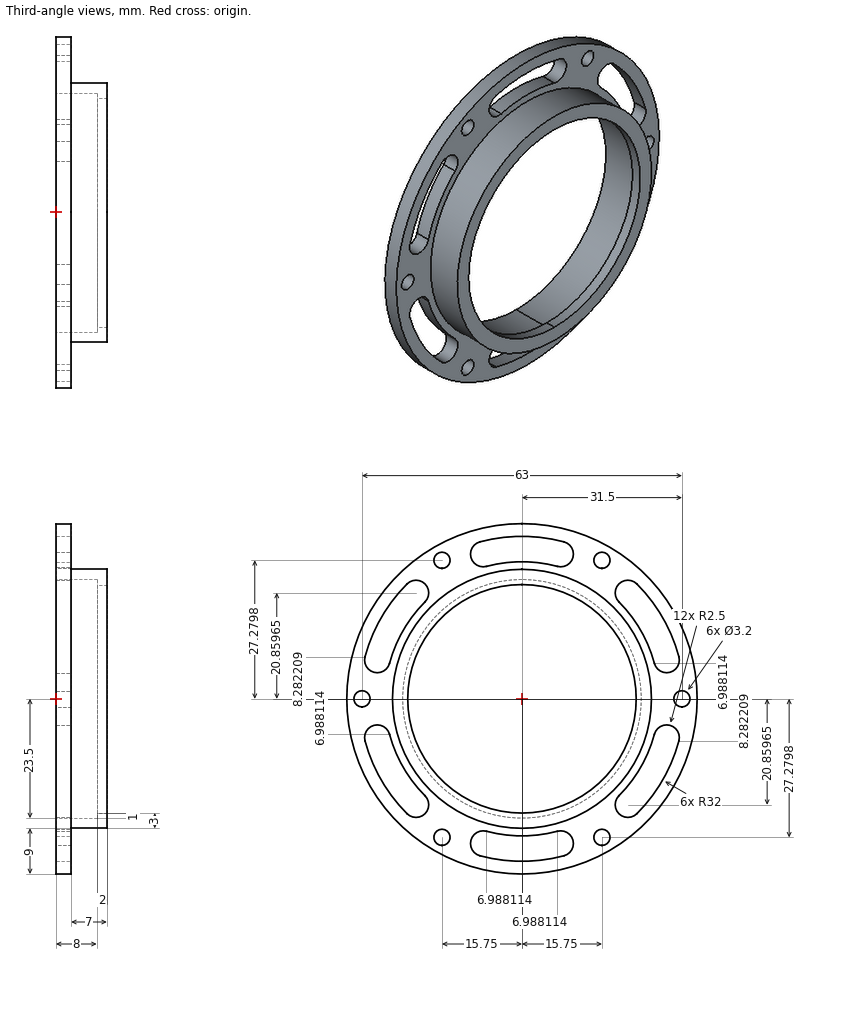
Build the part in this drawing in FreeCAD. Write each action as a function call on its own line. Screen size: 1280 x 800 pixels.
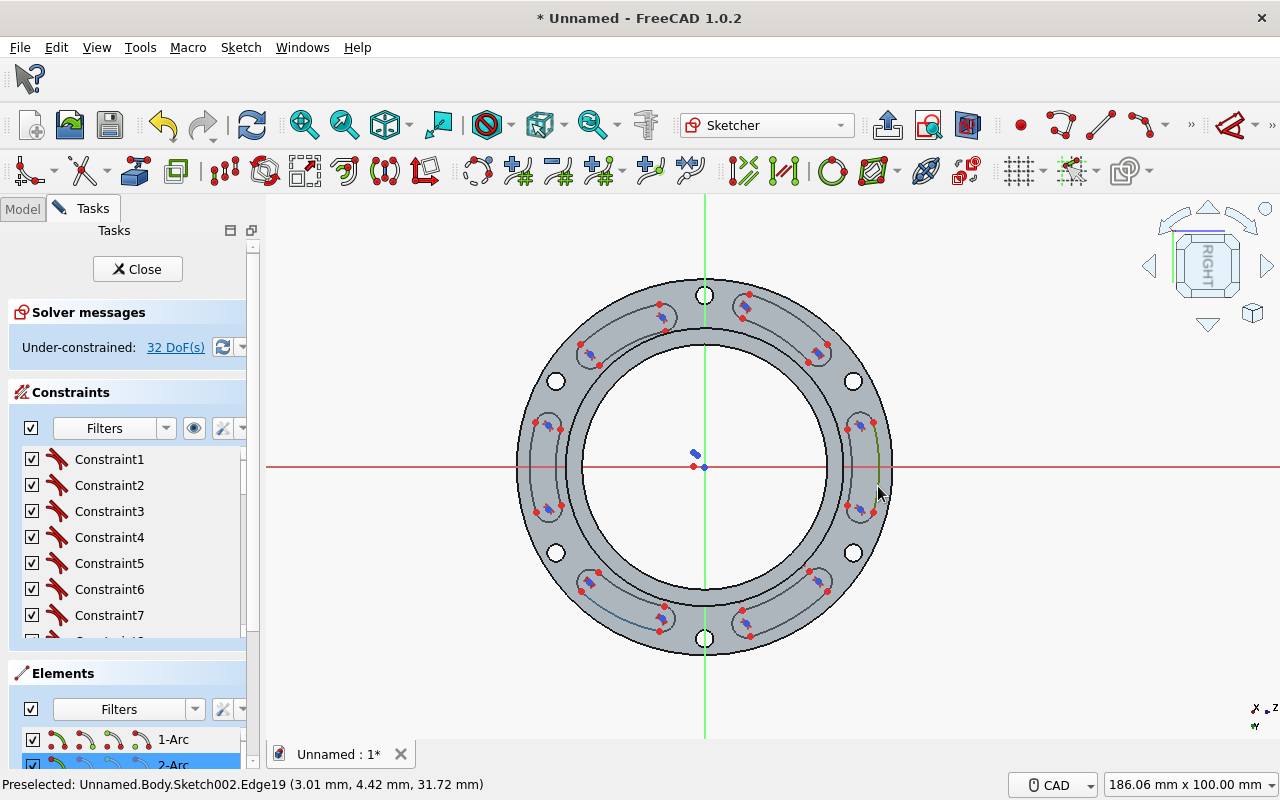
key(c)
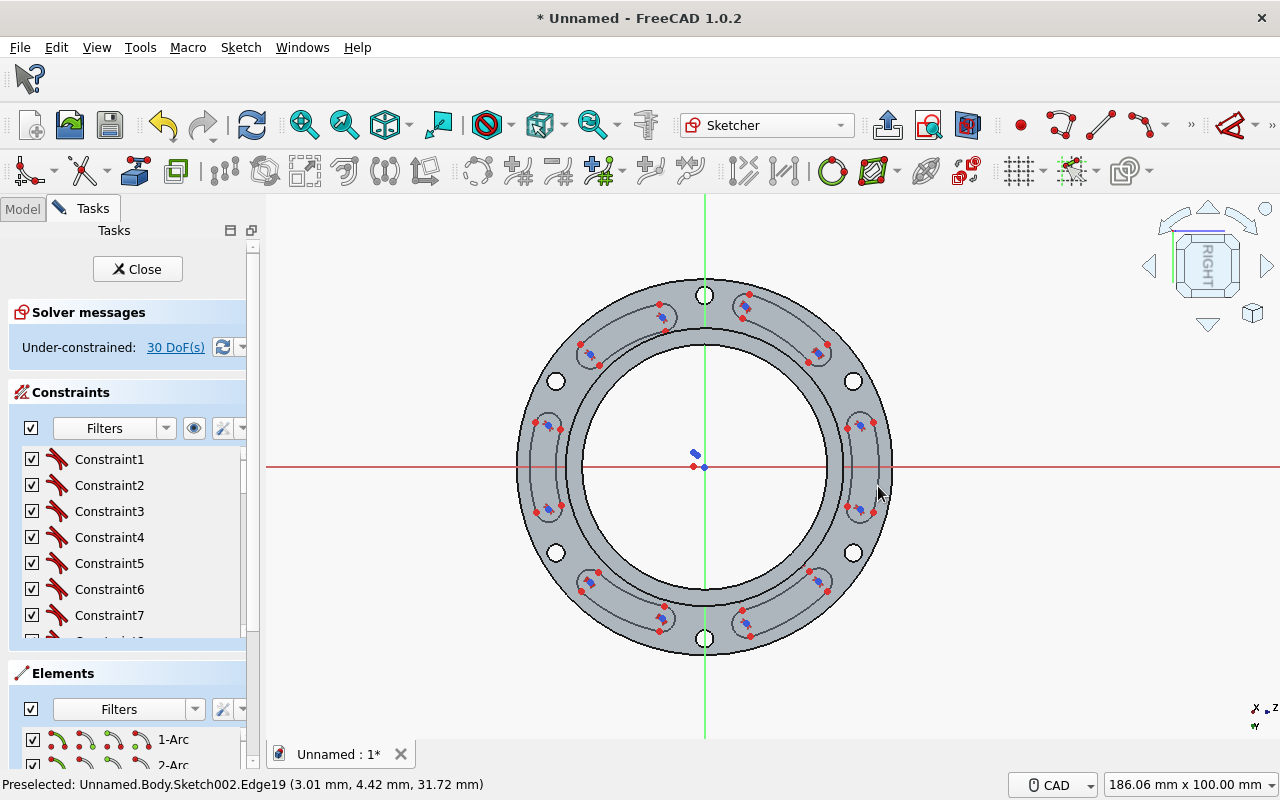
click(603, 608)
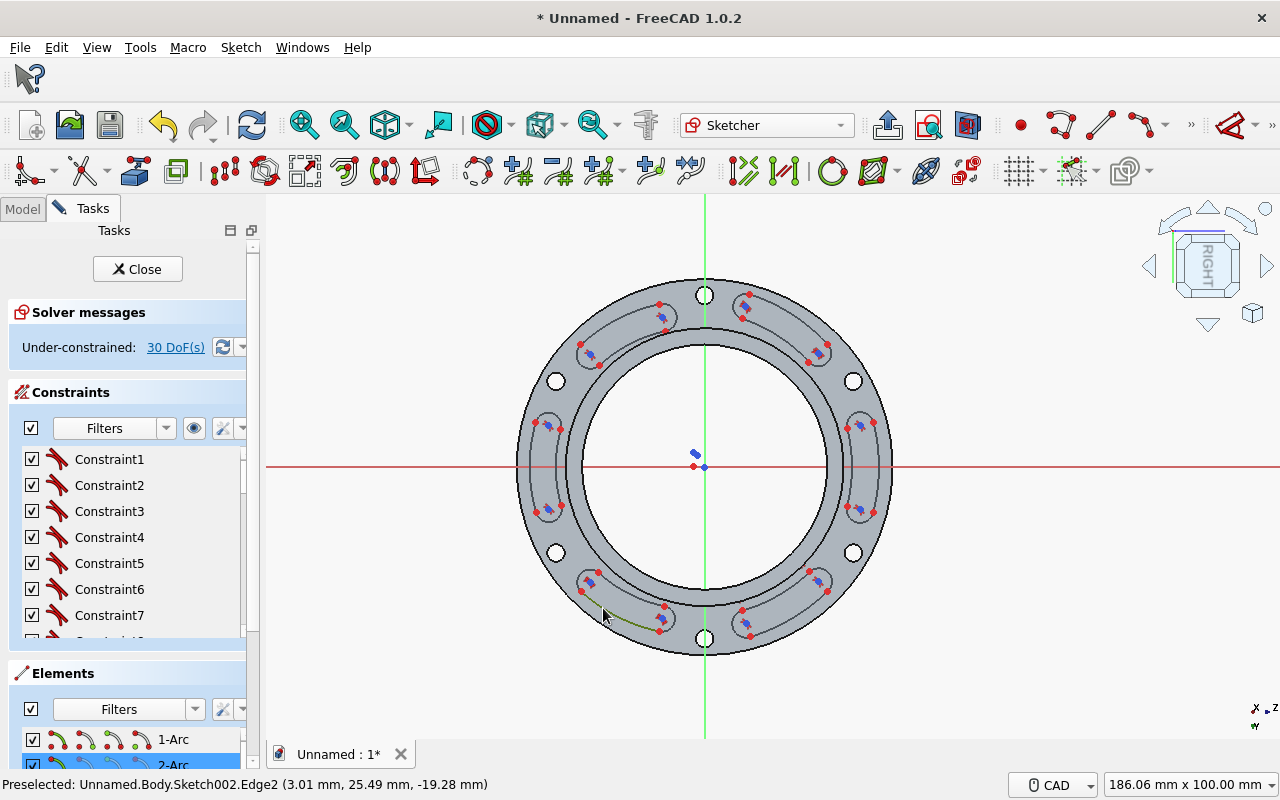
click(764, 603)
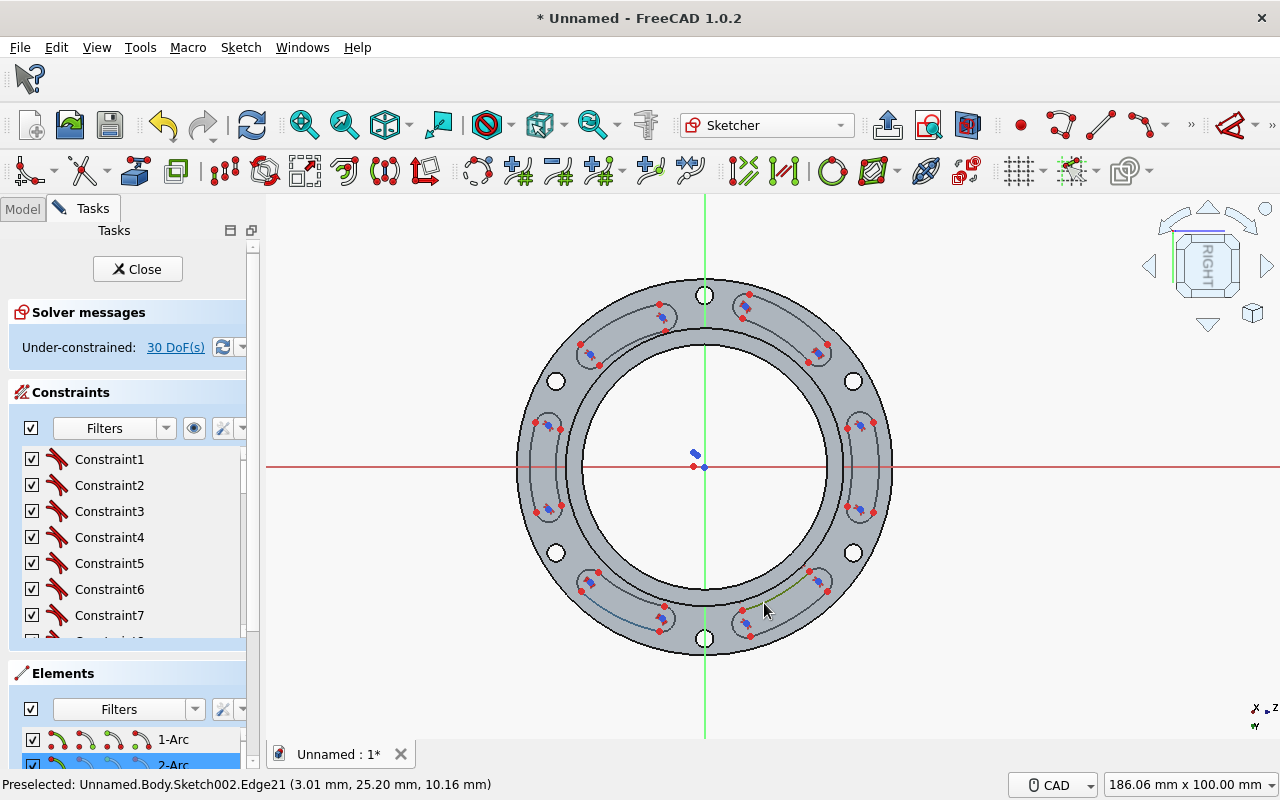
key(c)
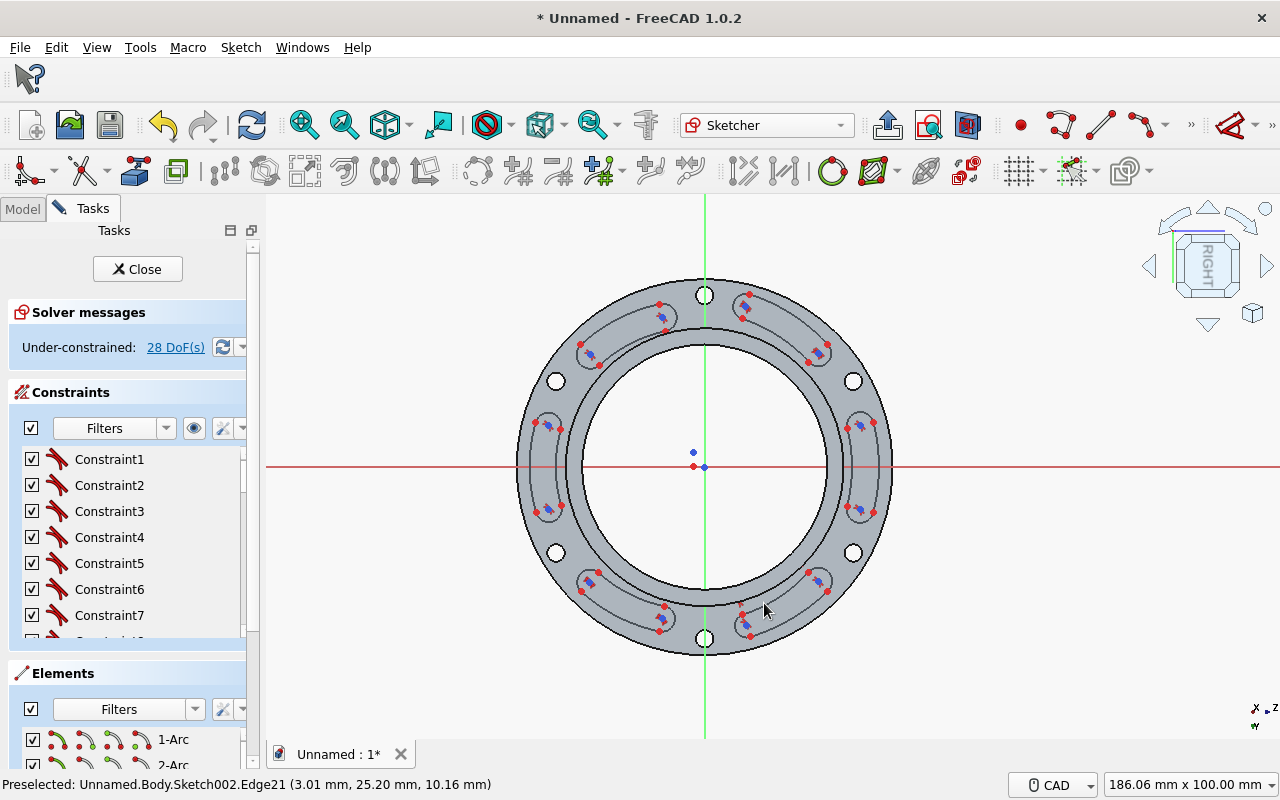
click(603, 608)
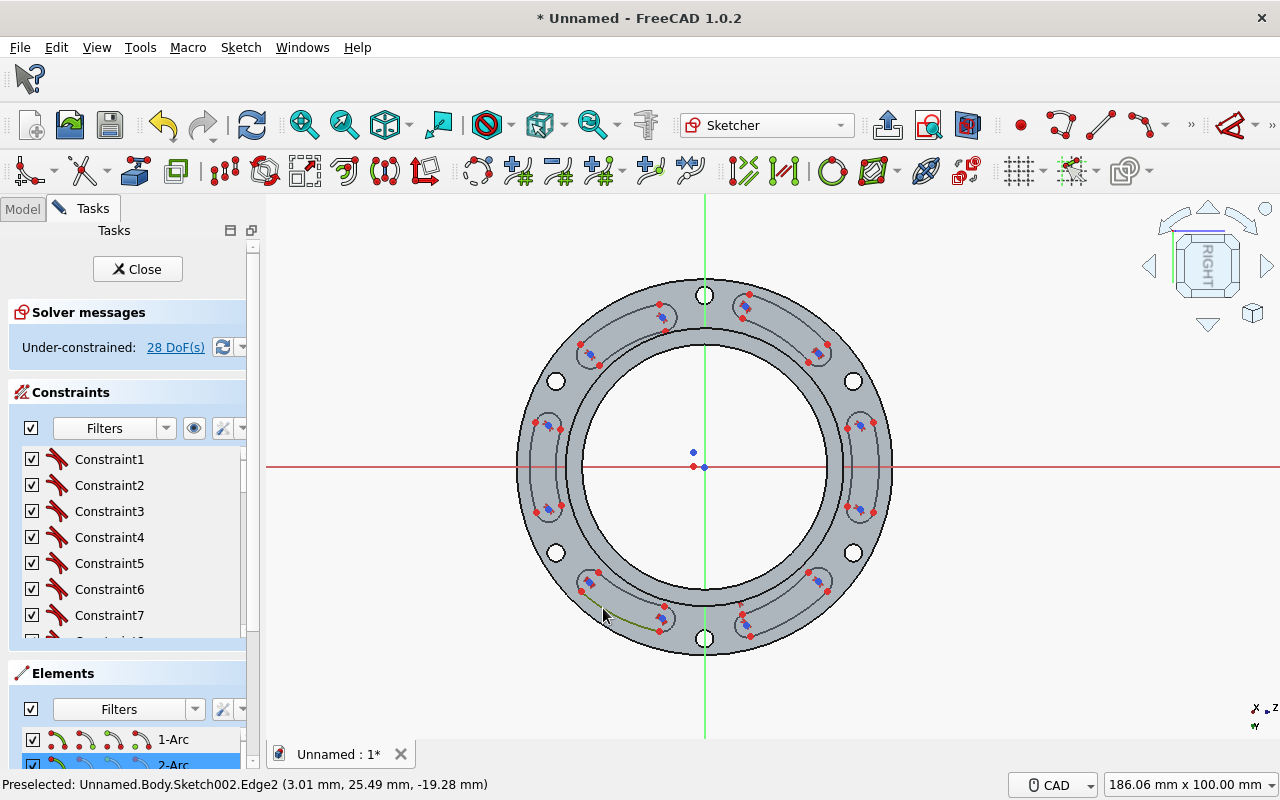
click(776, 627)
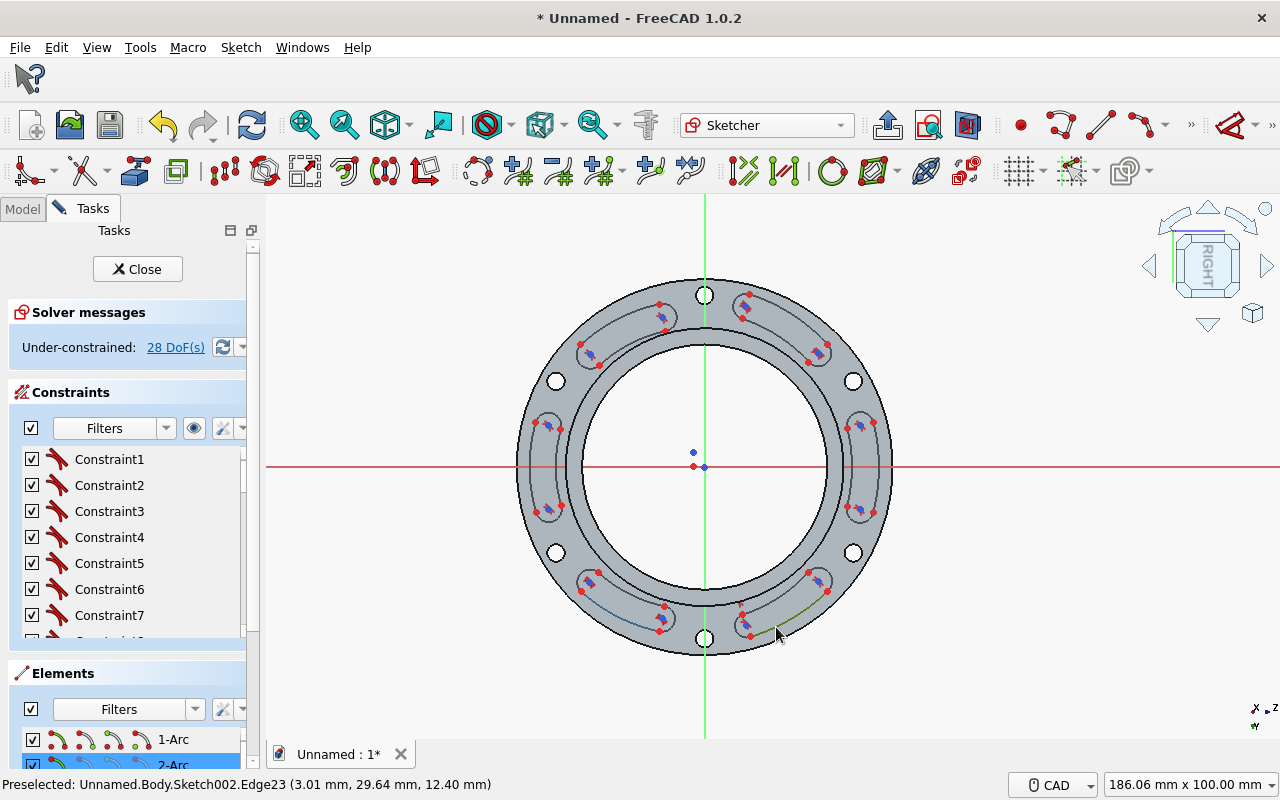
key(c)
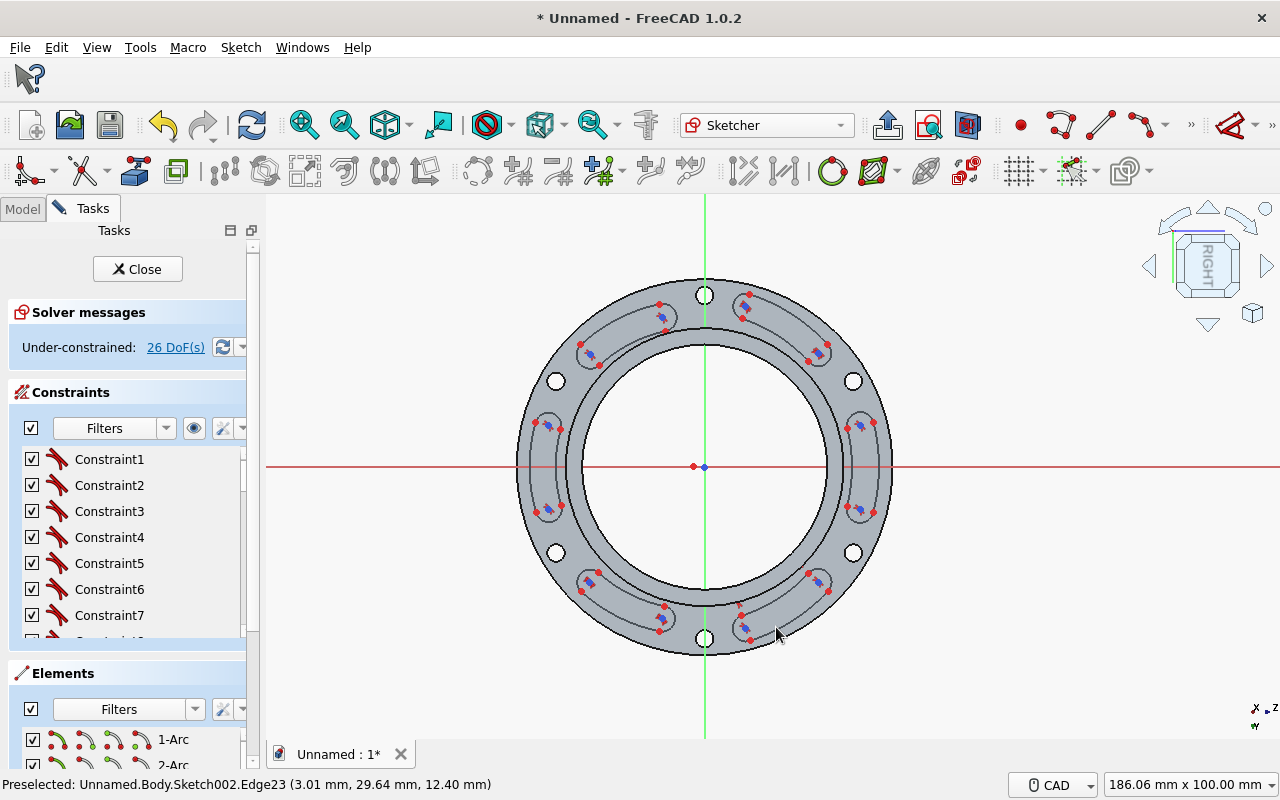
scroll(699, 467, up, 6)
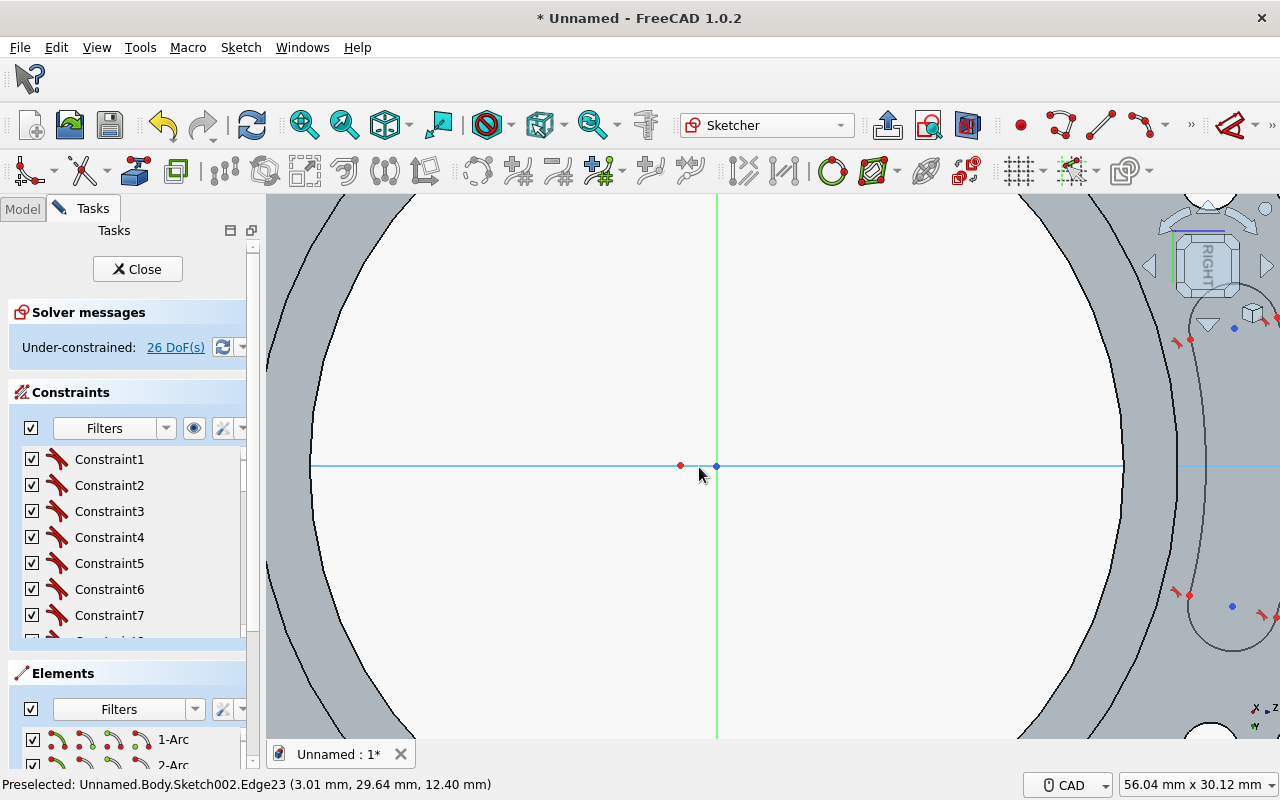
drag(671, 455, 727, 476)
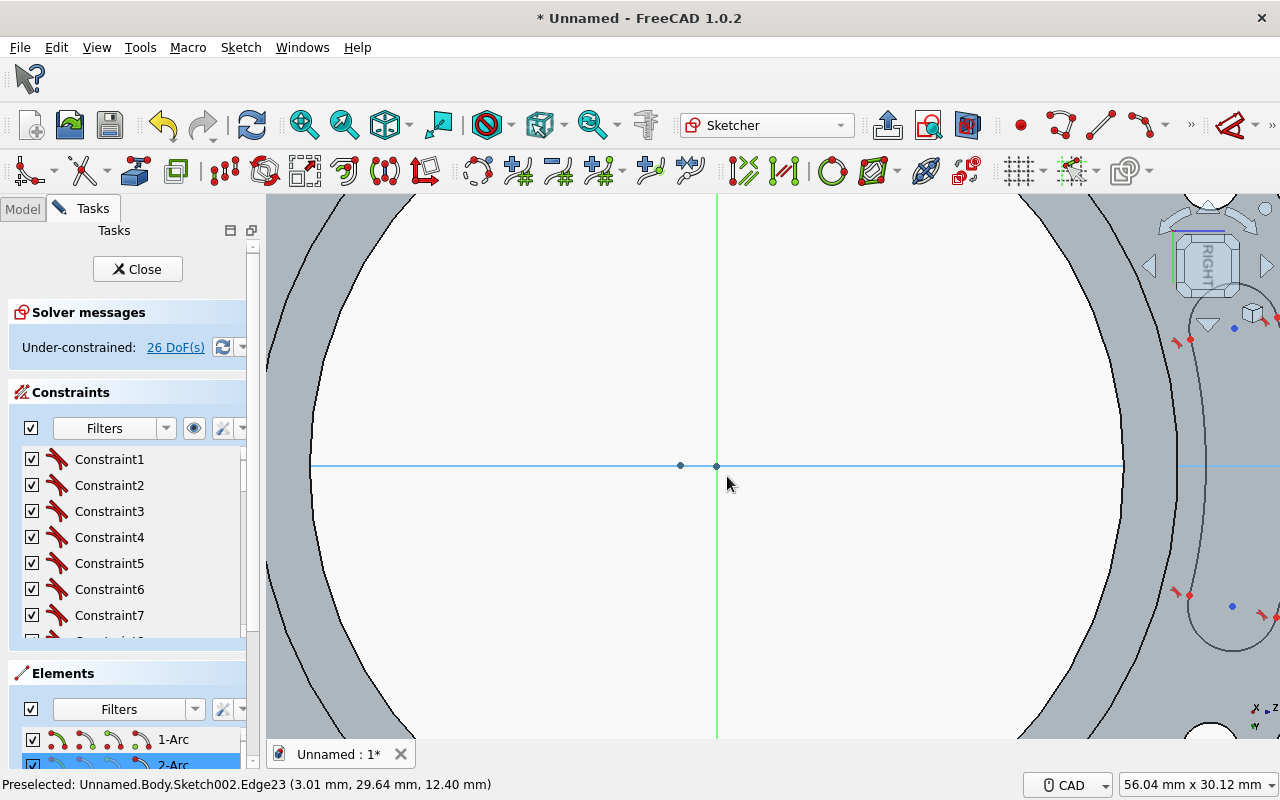
key(c)